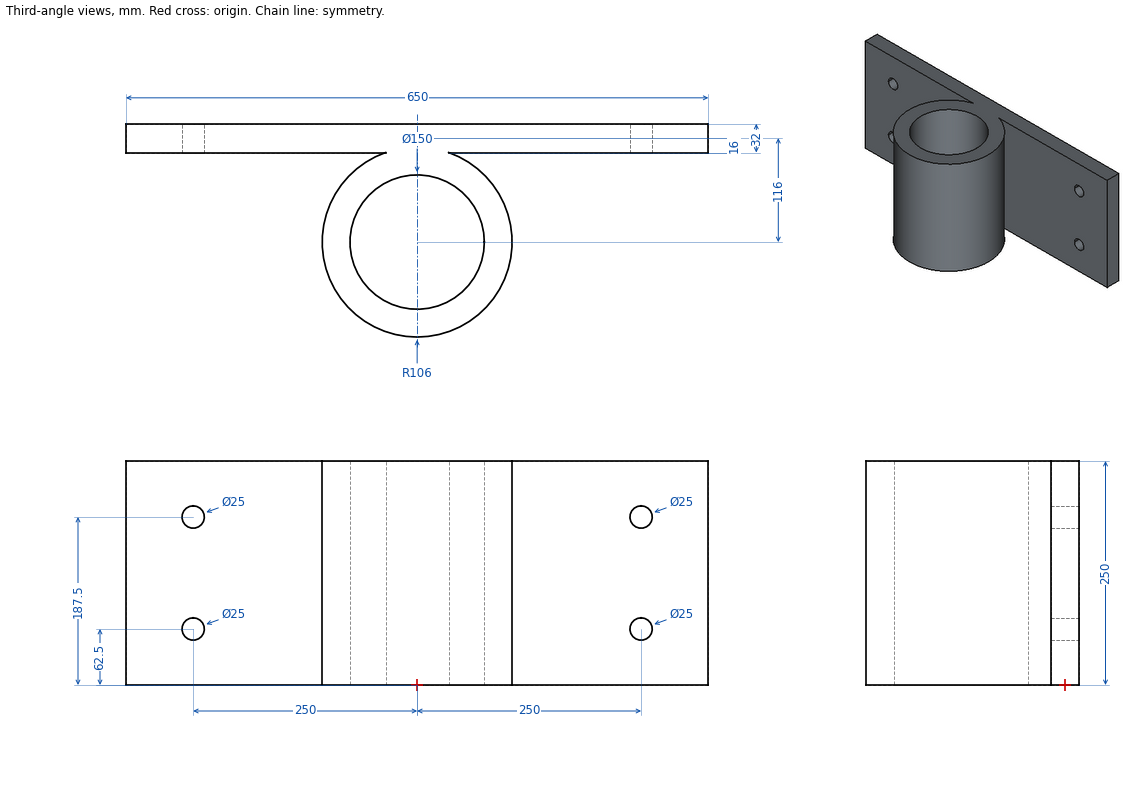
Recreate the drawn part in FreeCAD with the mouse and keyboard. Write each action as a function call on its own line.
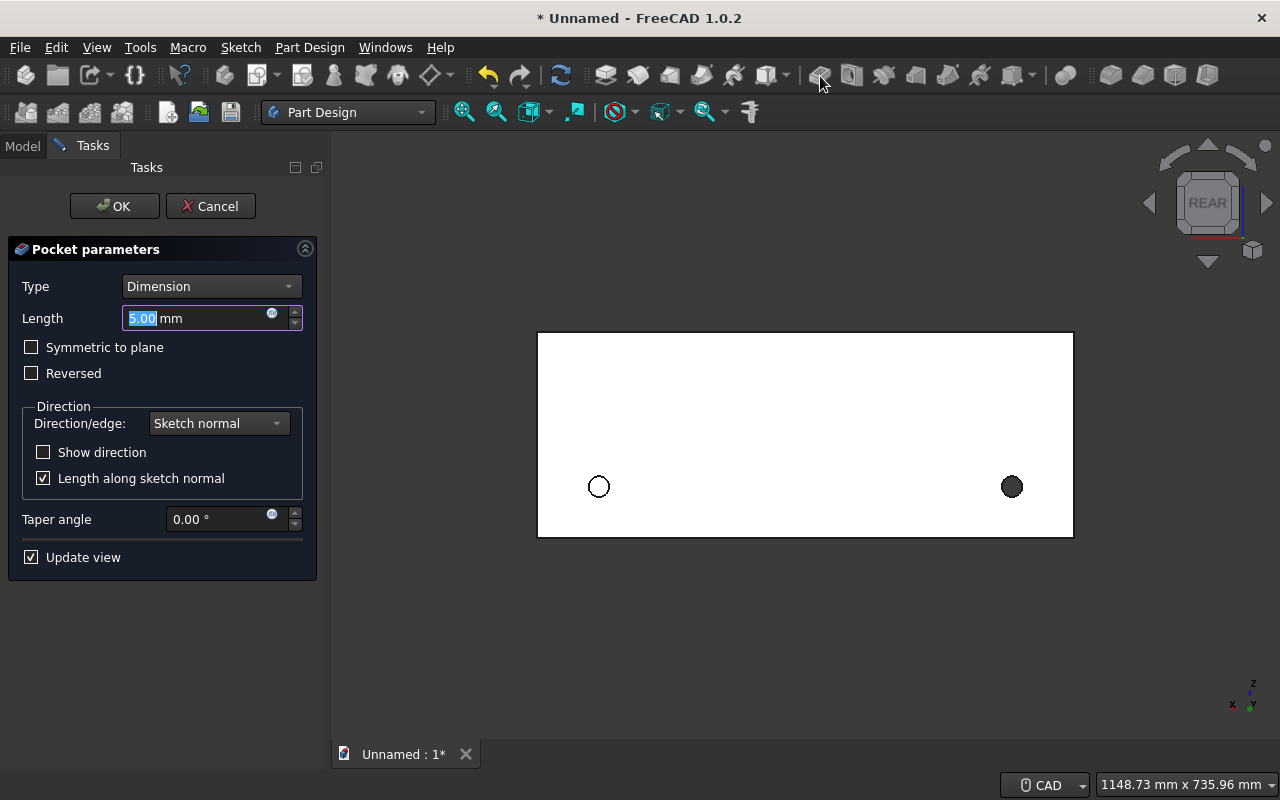
click(212, 286)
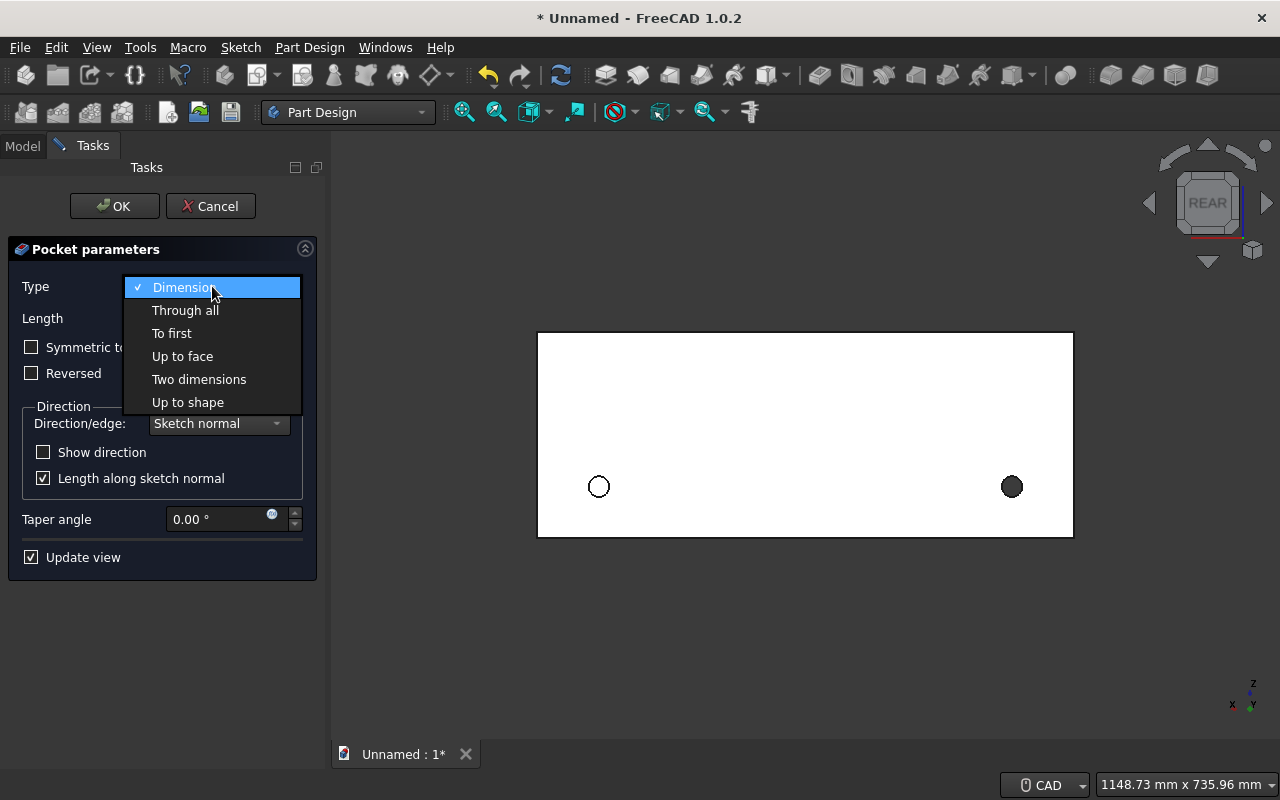
click(212, 334)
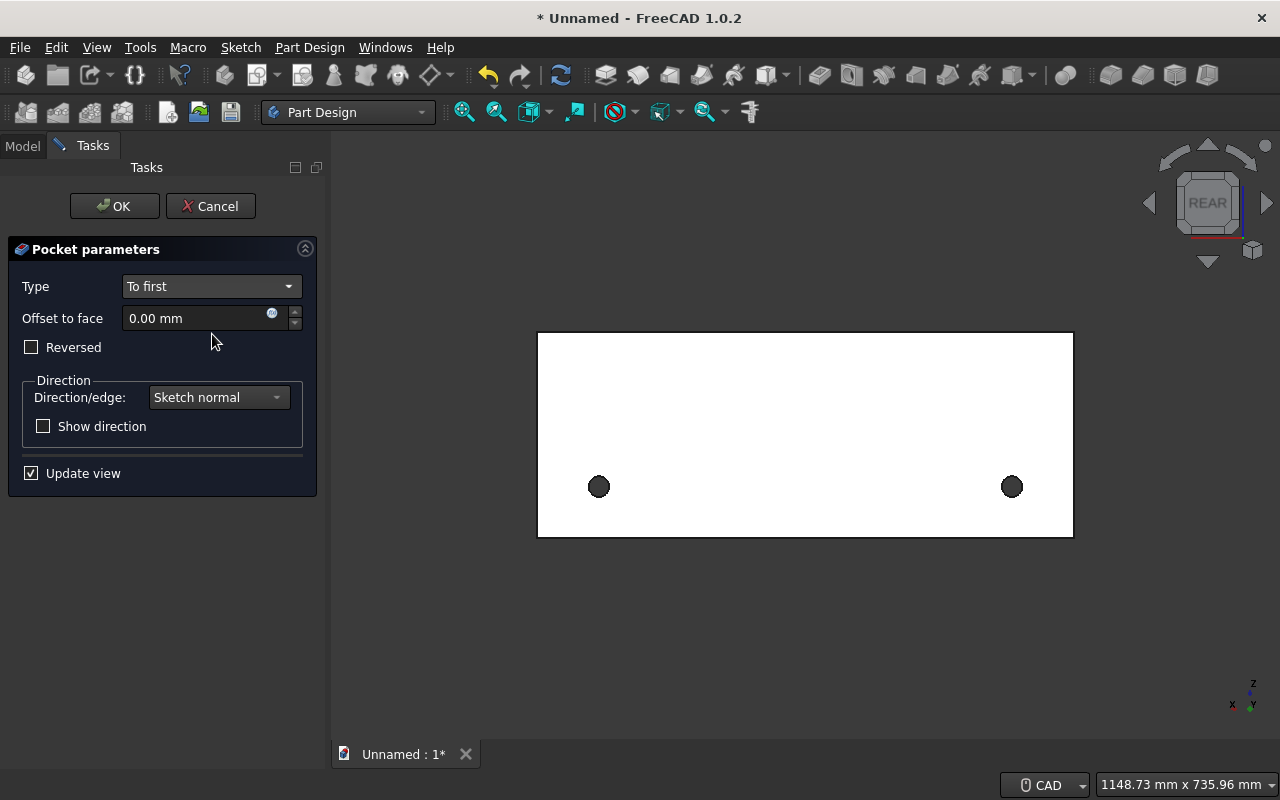
click(115, 206)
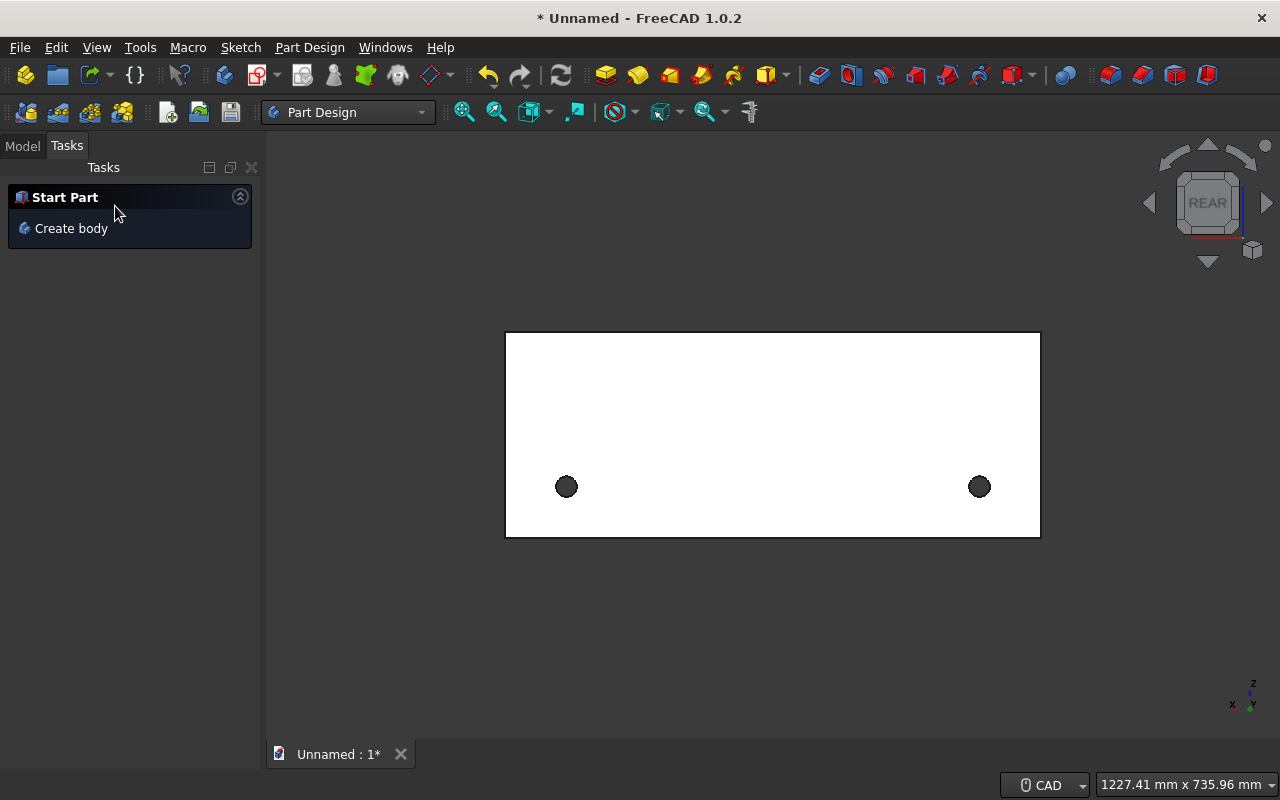
click(696, 434)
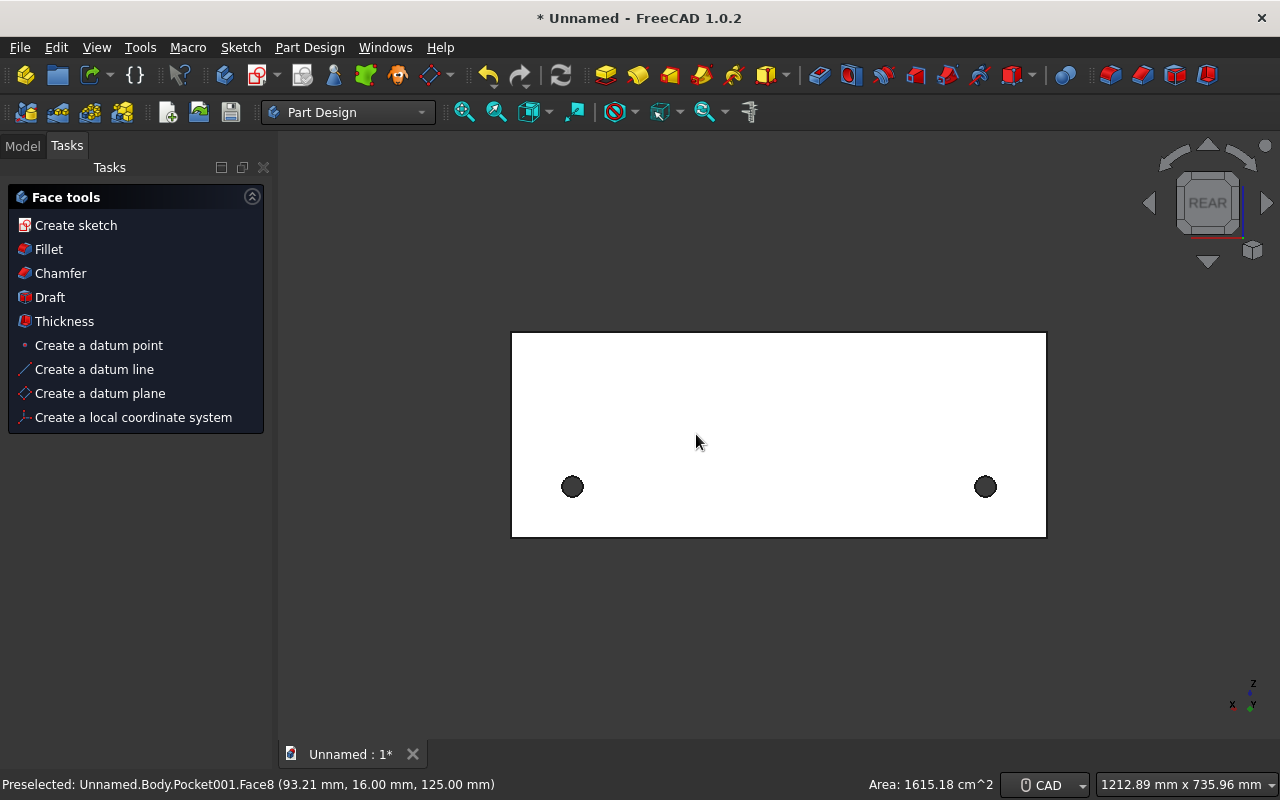
click(258, 76)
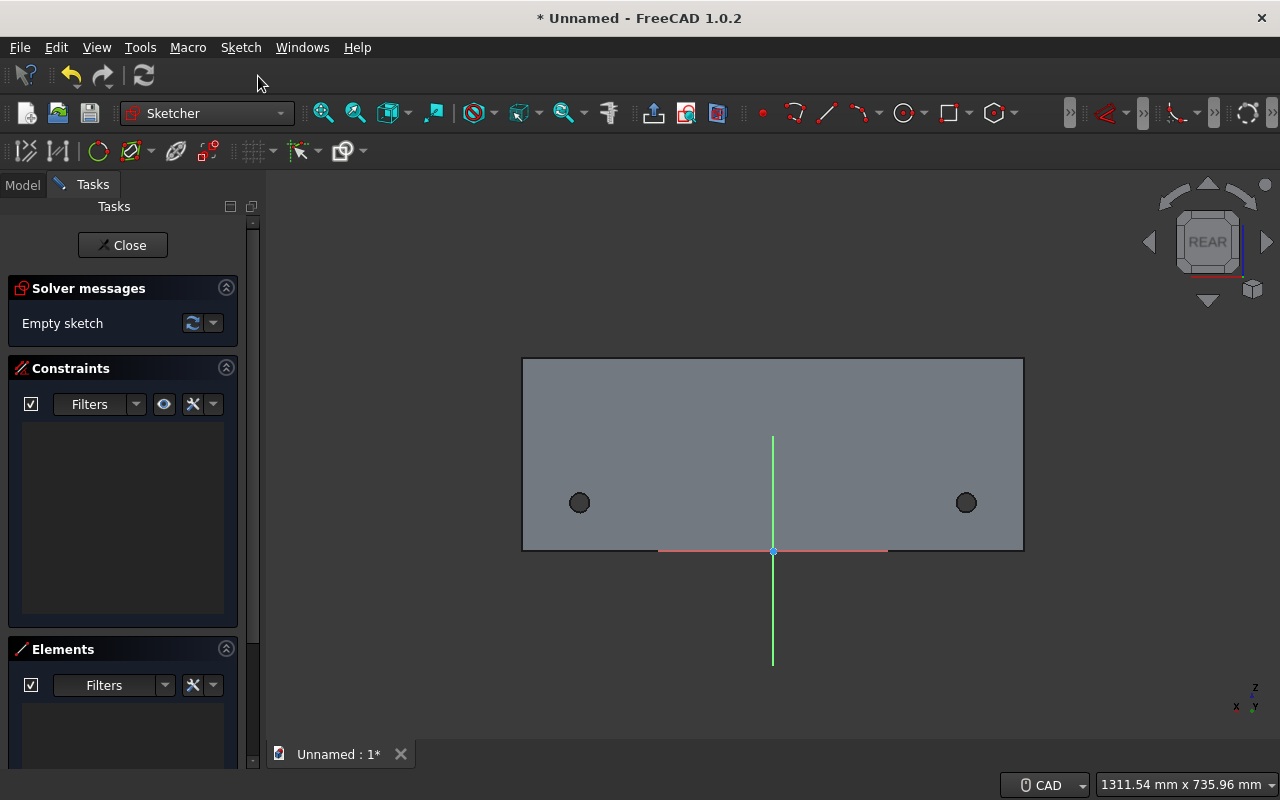
scroll(980, 404, up, 15)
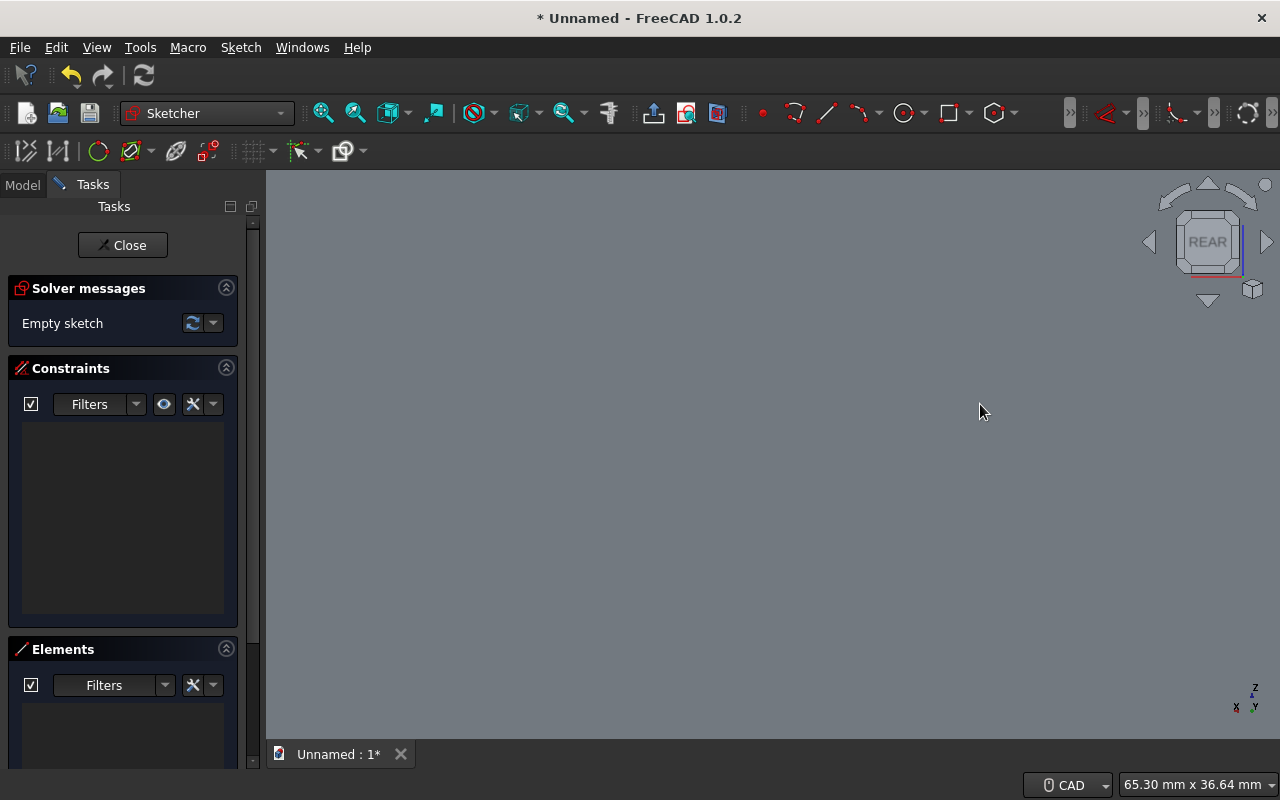
click(904, 114)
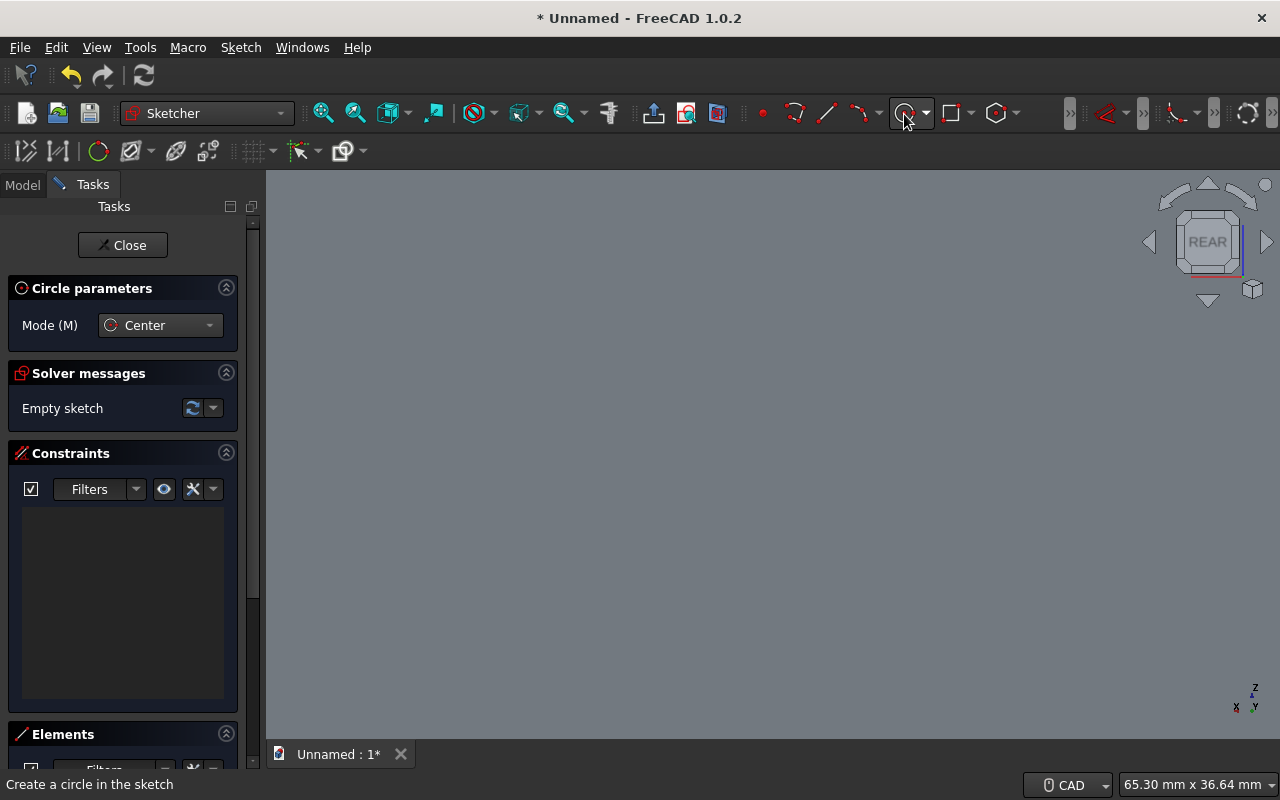
click(691, 440)
click(828, 303)
key(Escape)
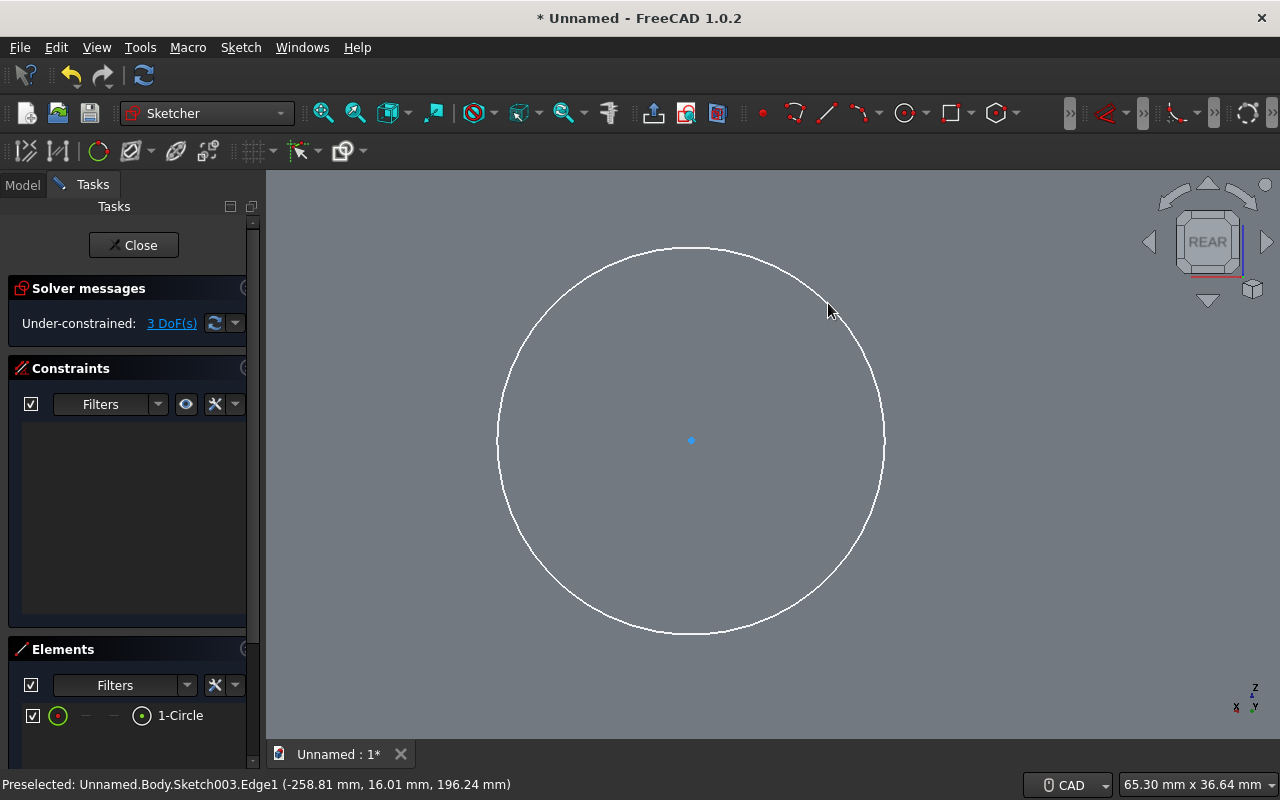
click(1106, 114)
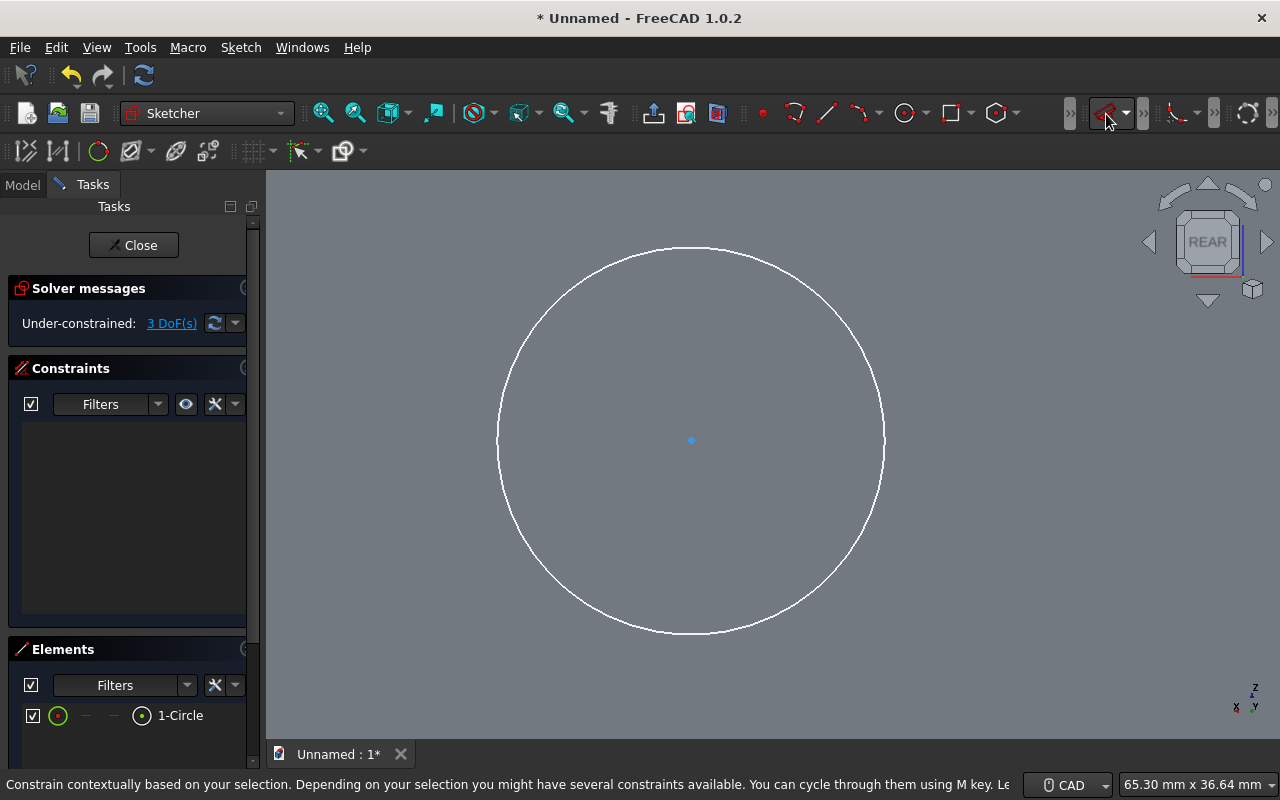
click(828, 304)
click(851, 281)